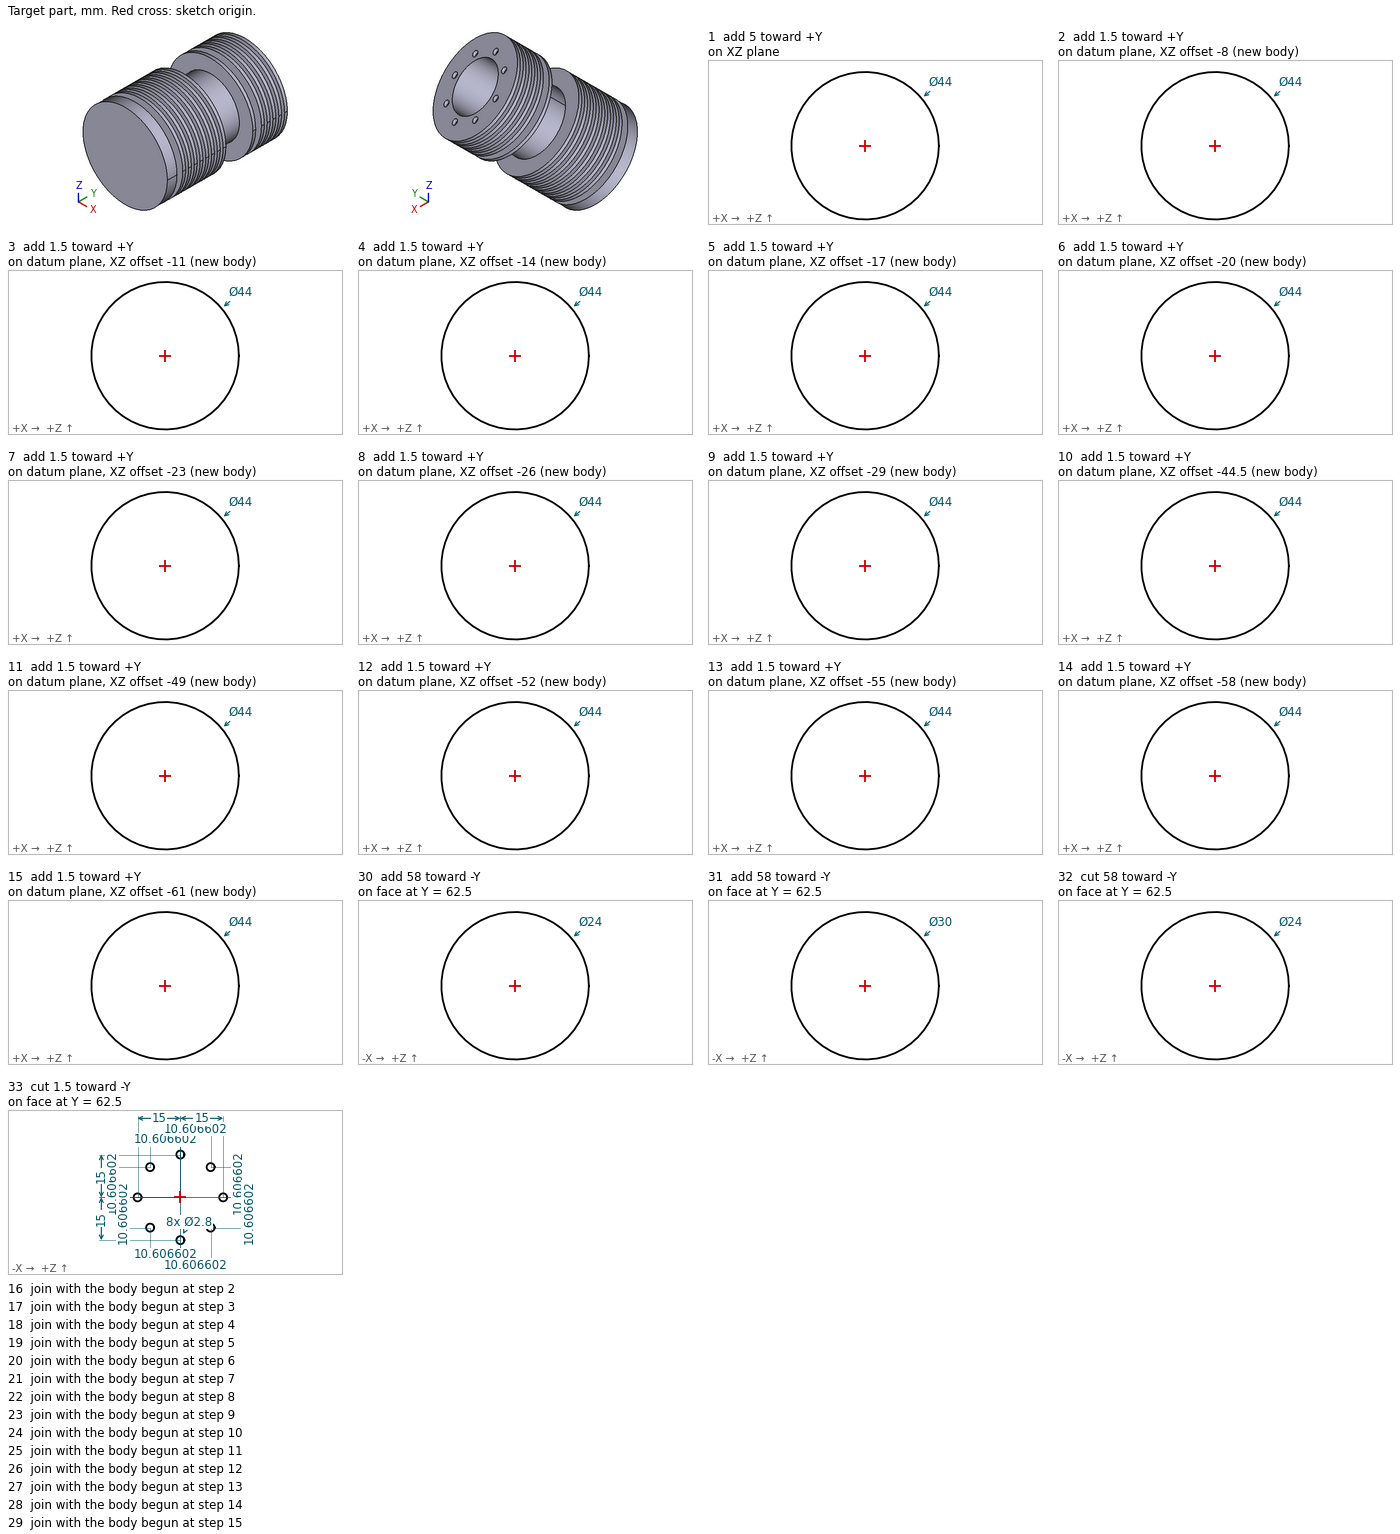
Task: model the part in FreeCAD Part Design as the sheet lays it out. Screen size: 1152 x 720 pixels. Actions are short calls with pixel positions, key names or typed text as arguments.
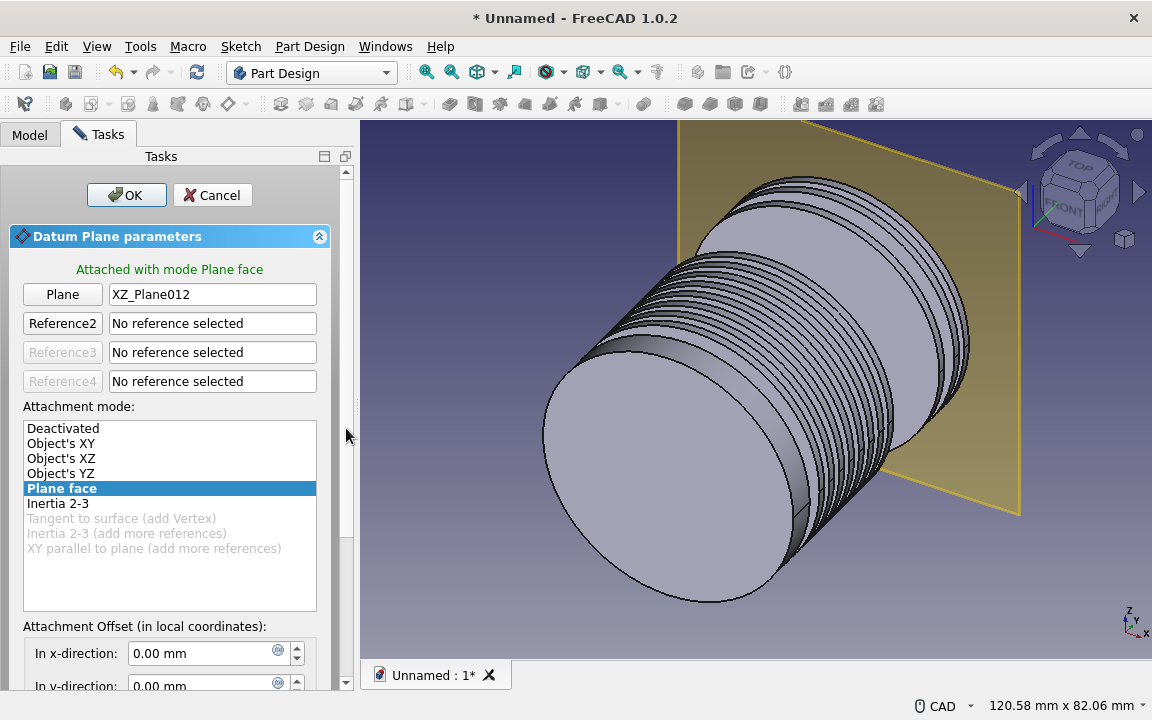
click(127, 195)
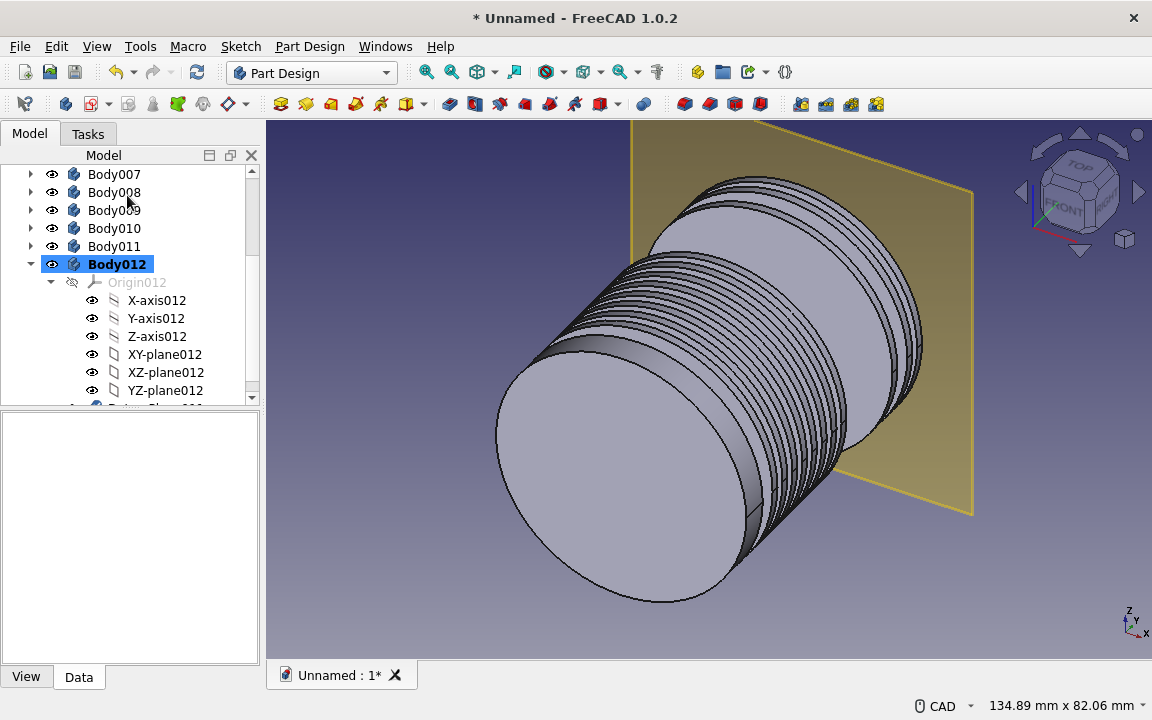
scroll(121, 278, down, 3)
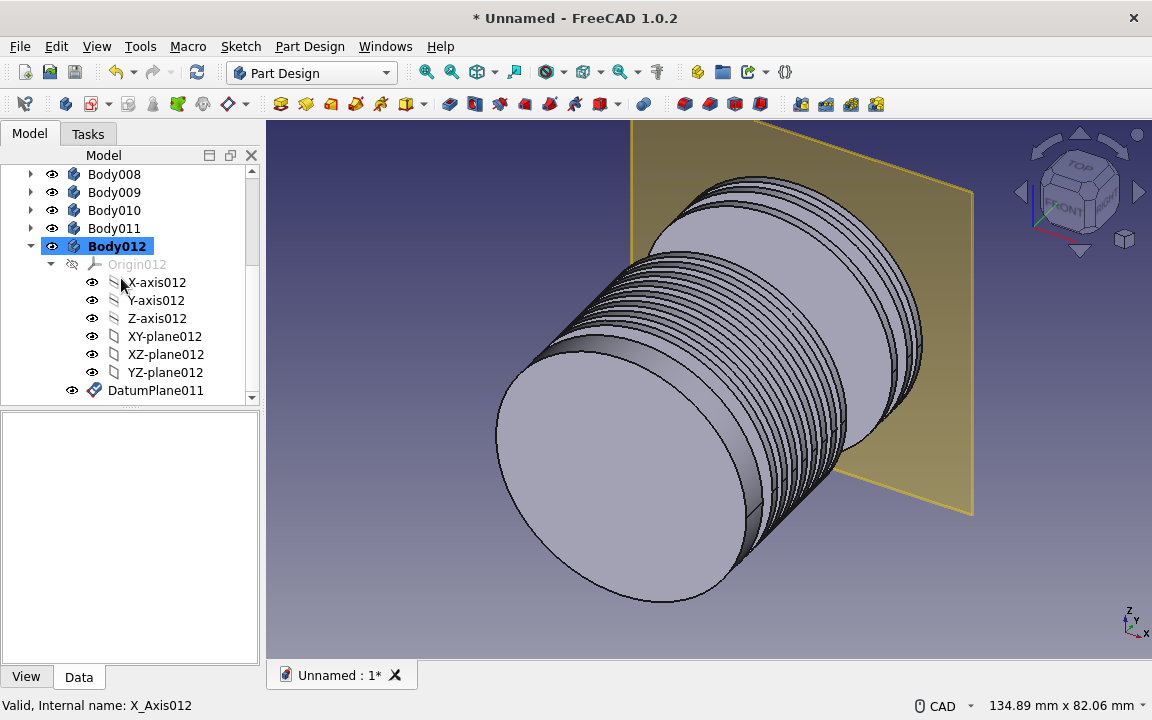
click(117, 390)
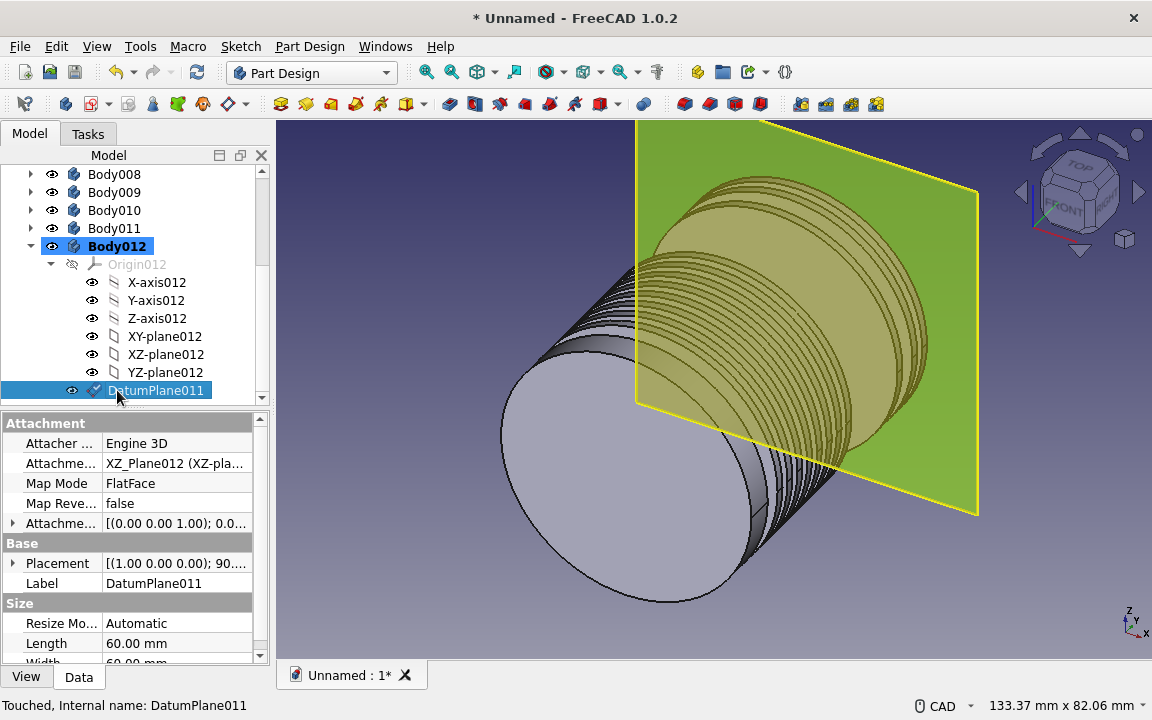
click(90, 104)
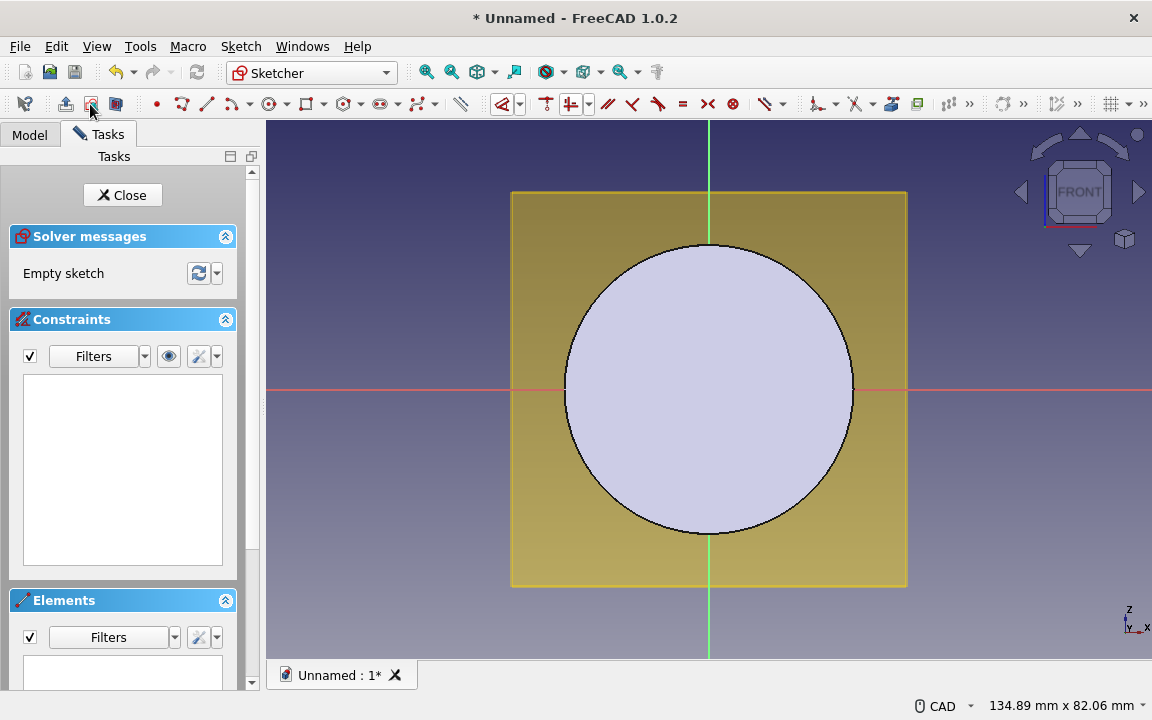
click(268, 104)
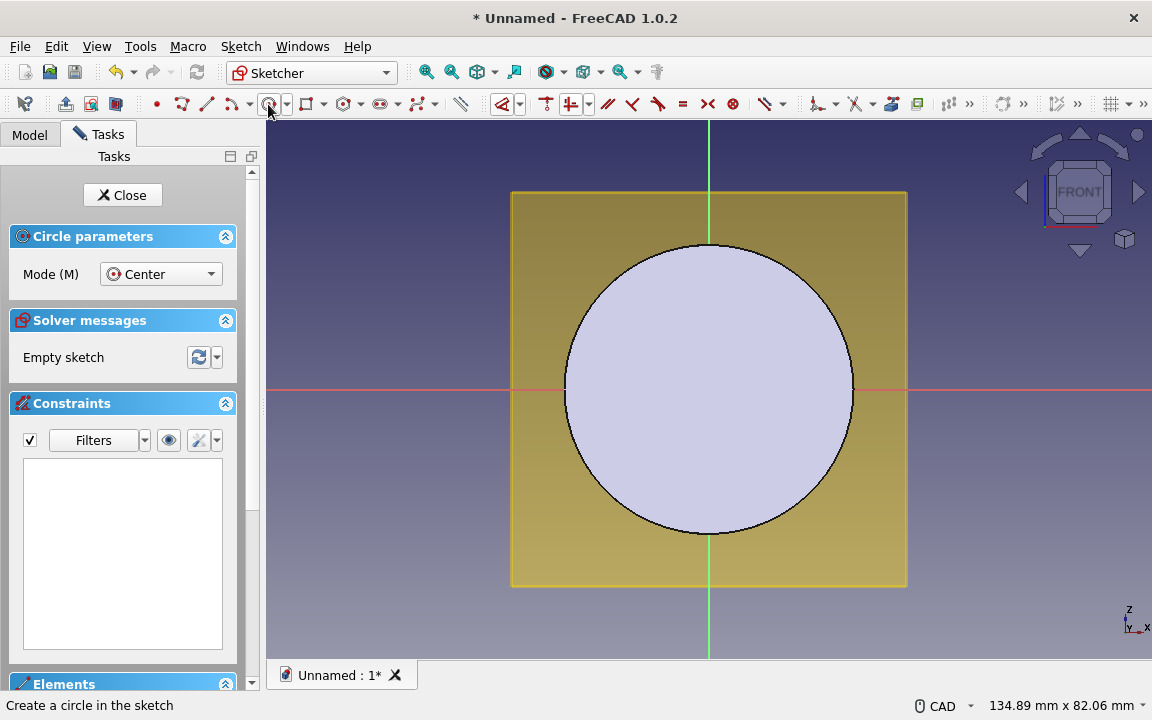
click(709, 390)
click(811, 287)
key(Escape)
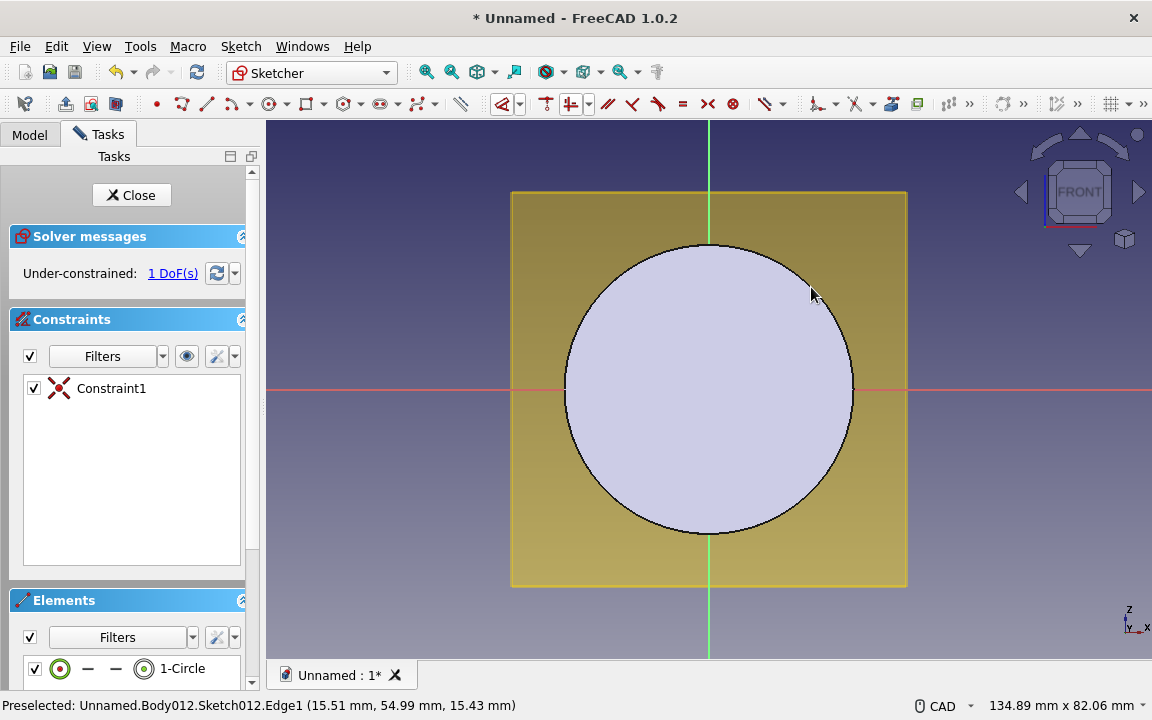
click(810, 287)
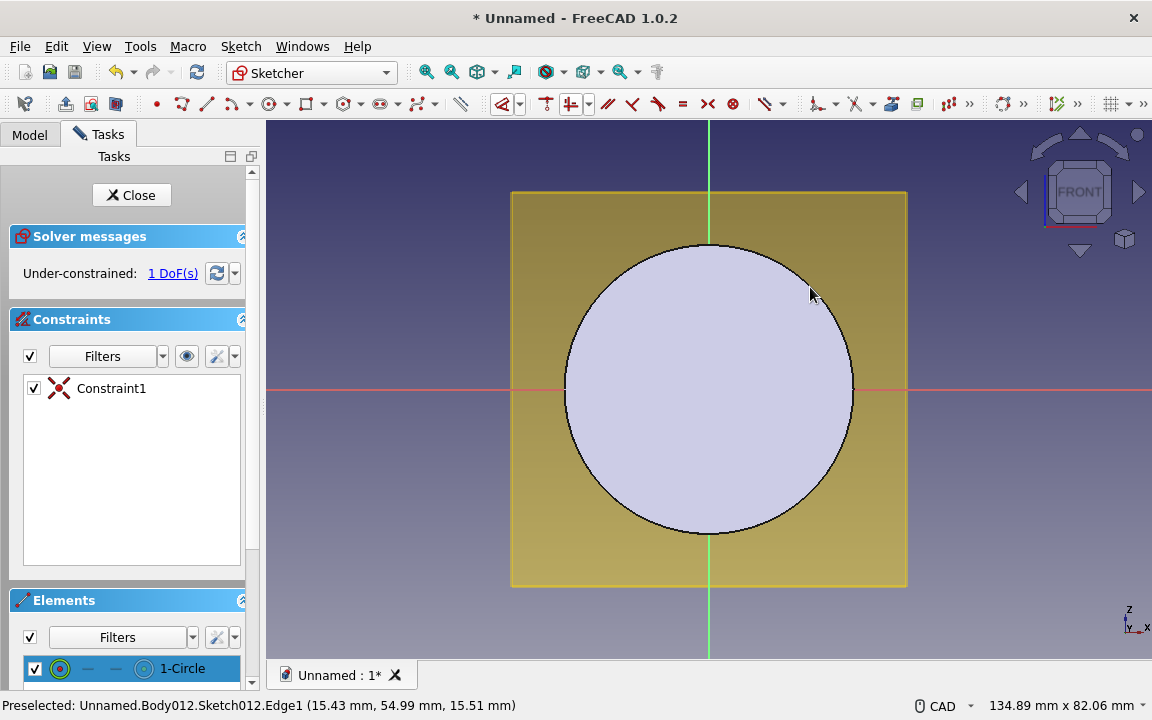
key(k)
key(o)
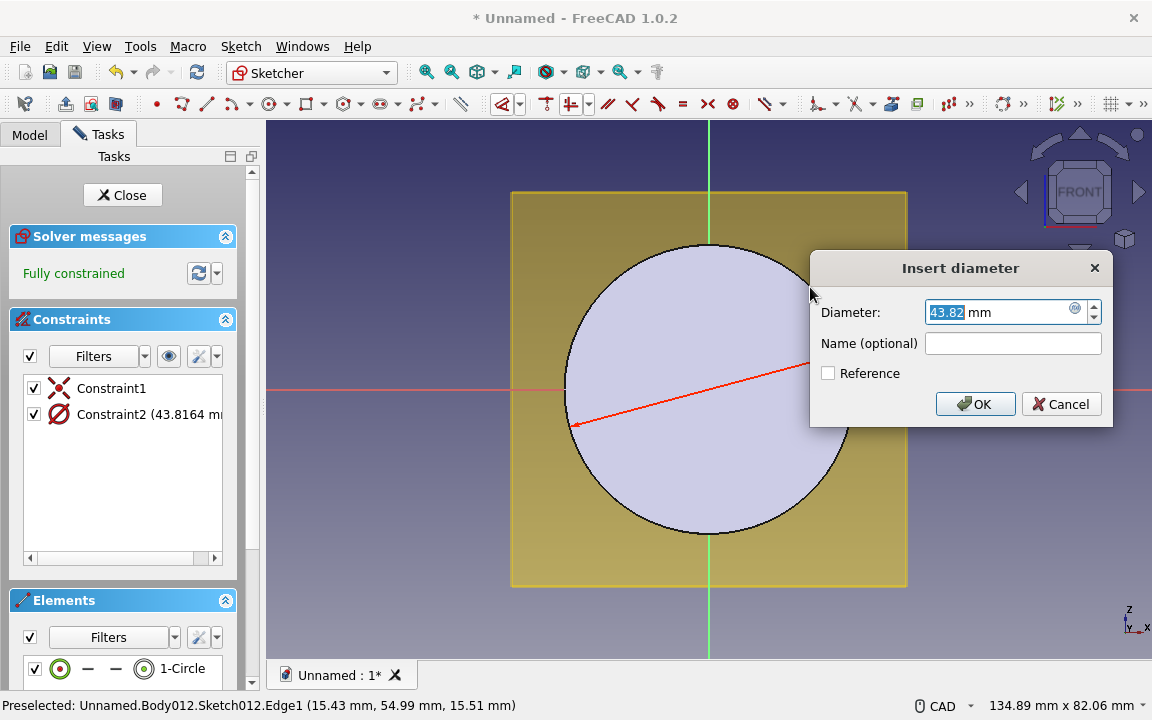
text(44)
key(Return)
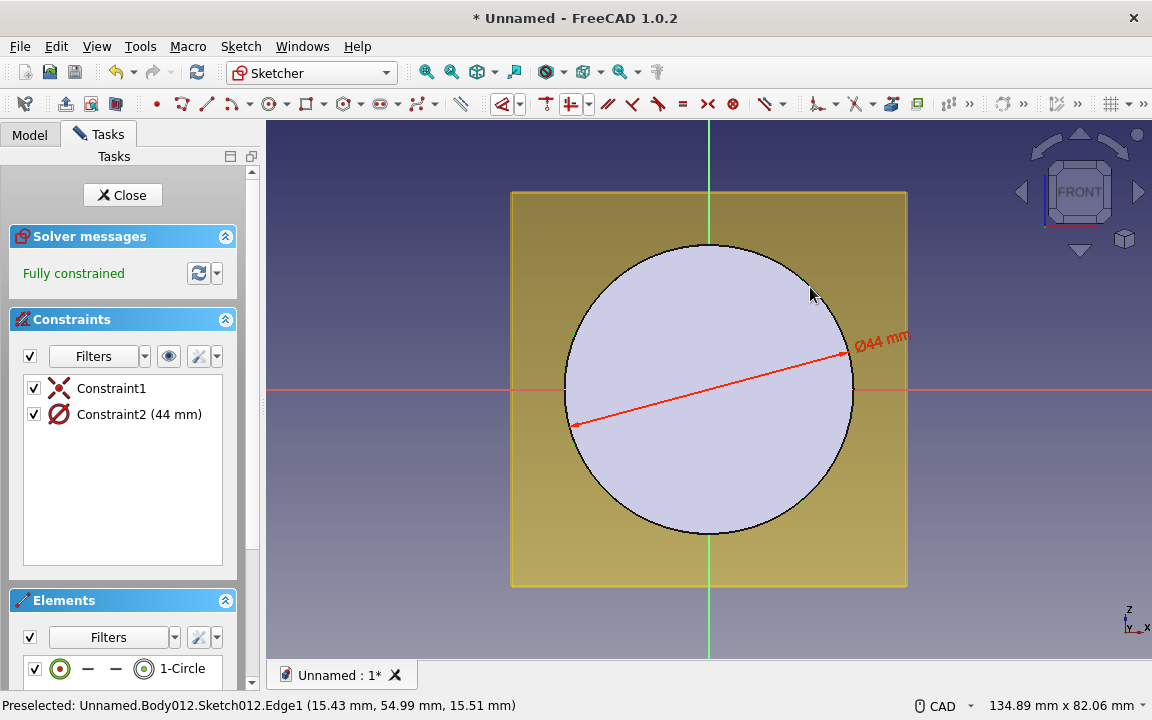
click(123, 195)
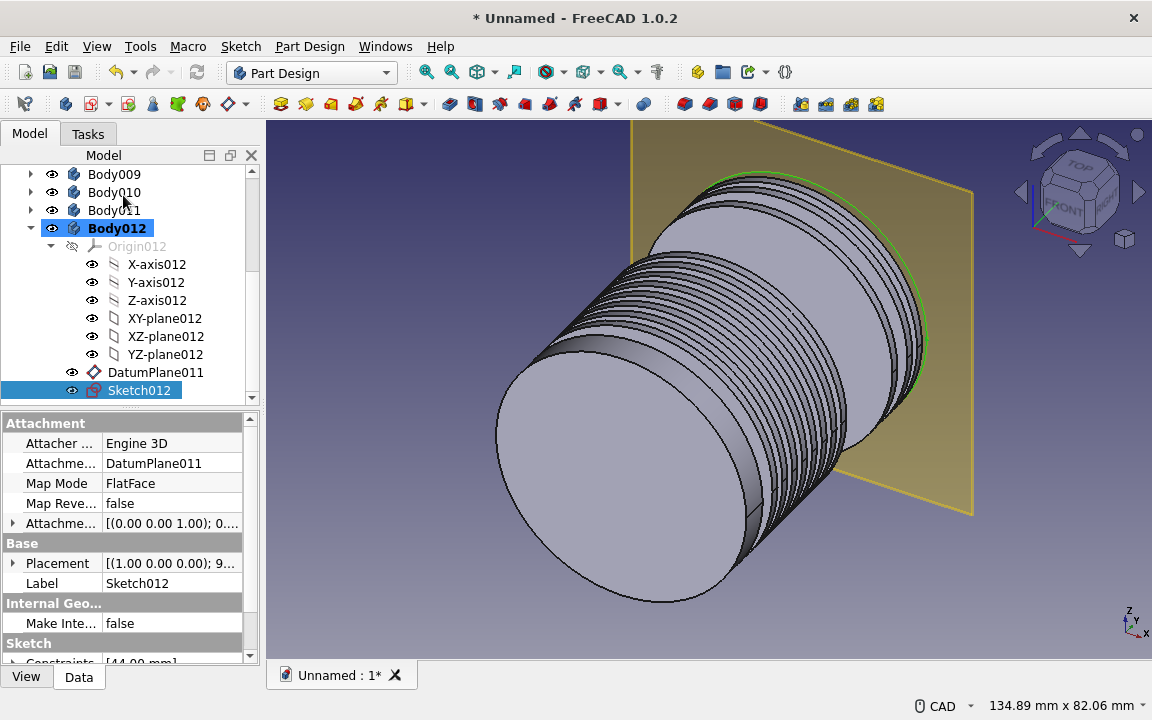
click(281, 104)